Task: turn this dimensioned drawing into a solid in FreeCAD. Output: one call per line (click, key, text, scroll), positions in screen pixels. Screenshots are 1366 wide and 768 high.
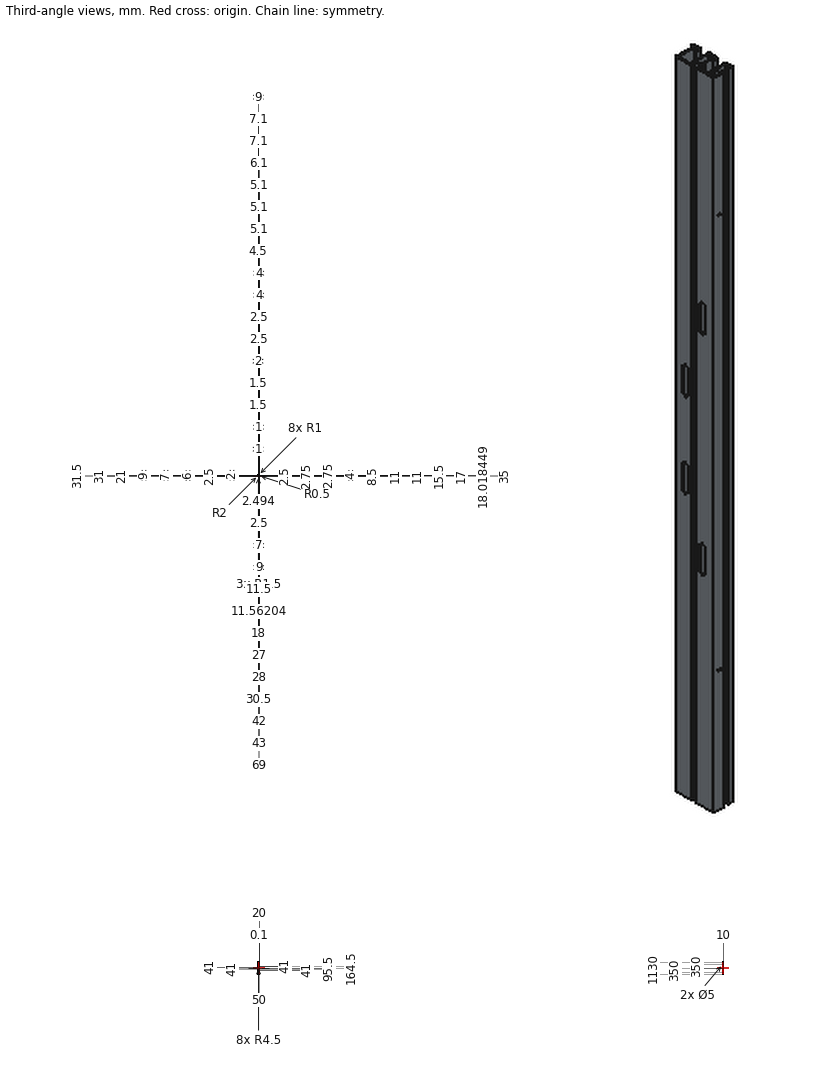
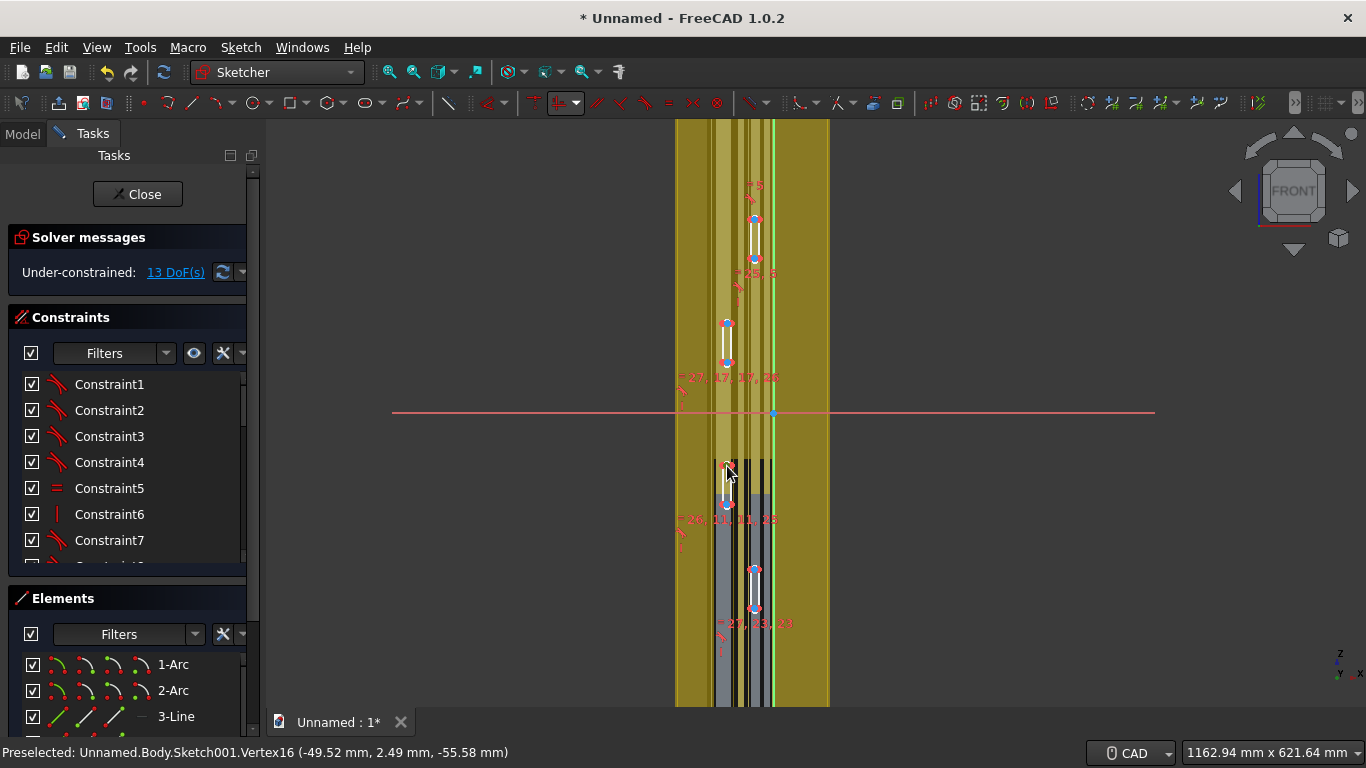
scroll(727, 363, up, 6)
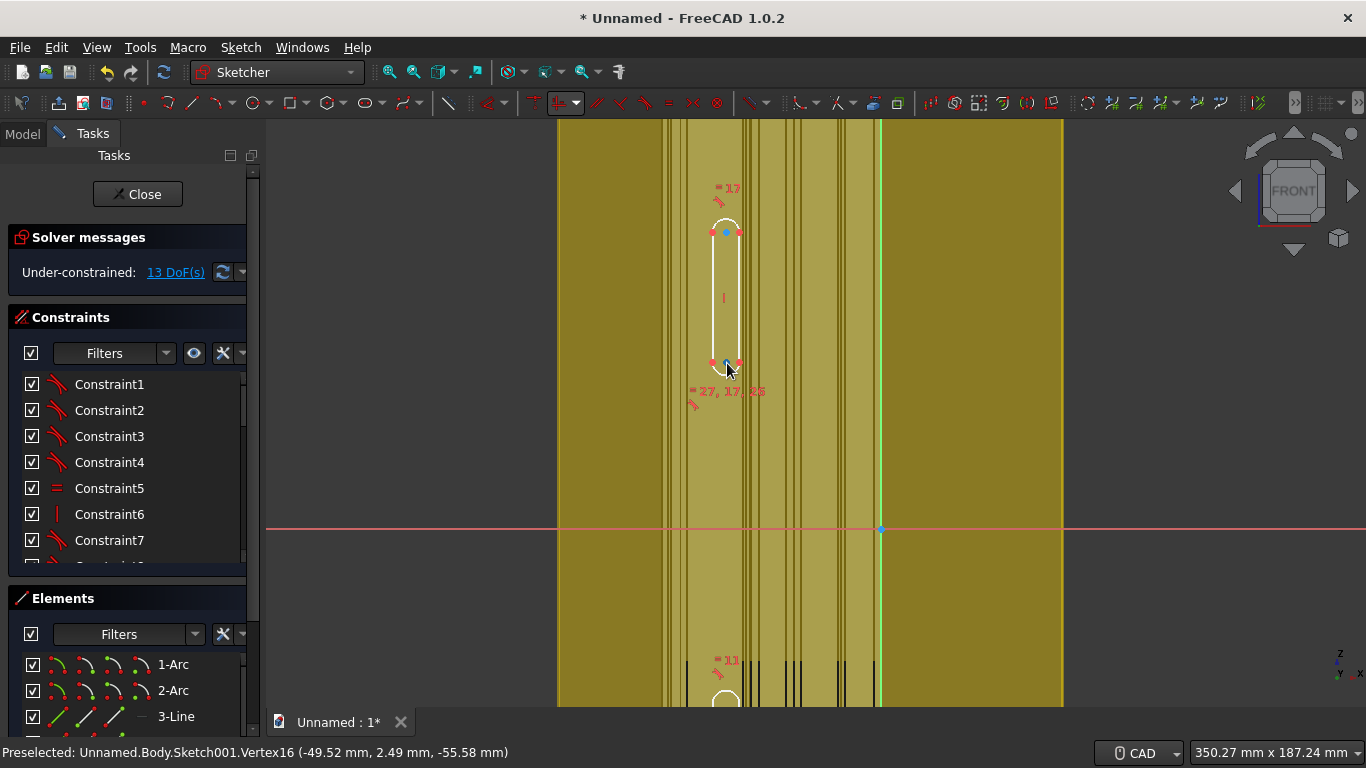
click(726, 362)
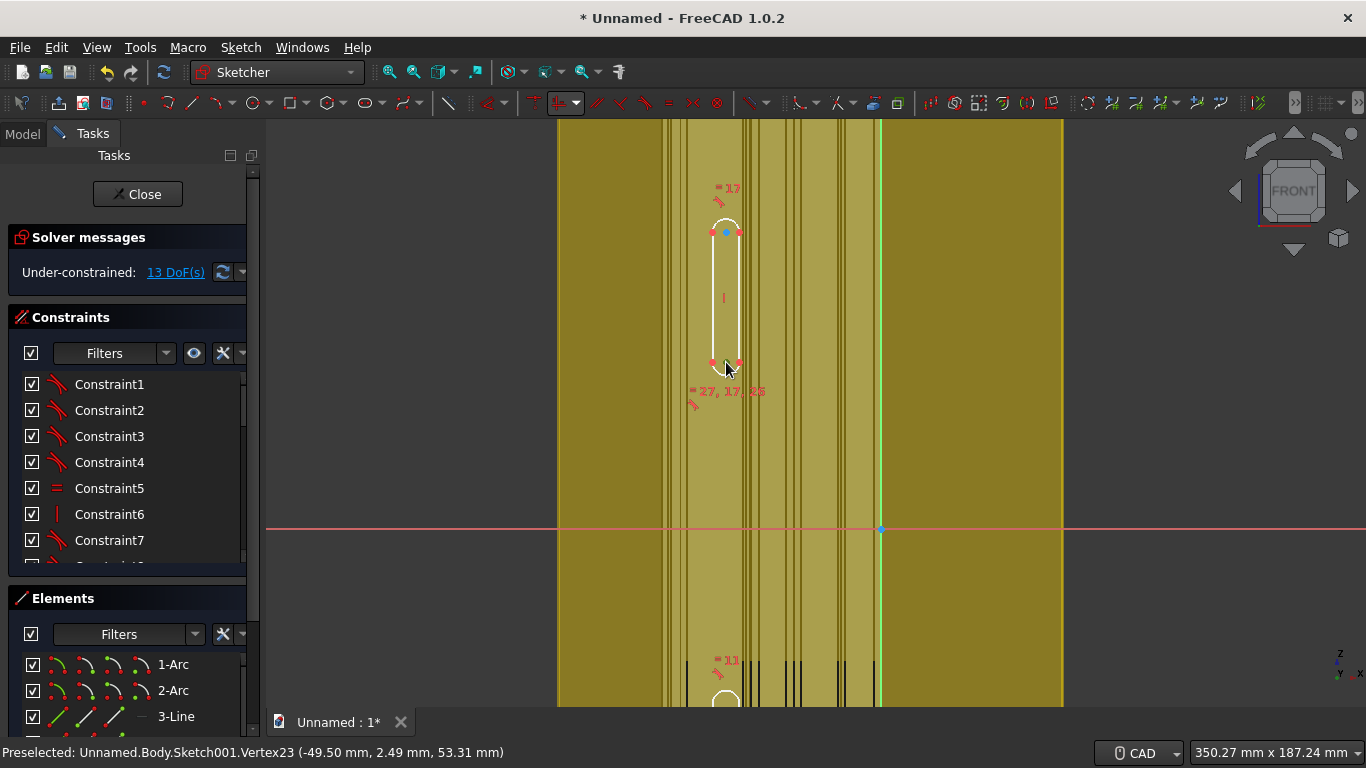
click(359, 529)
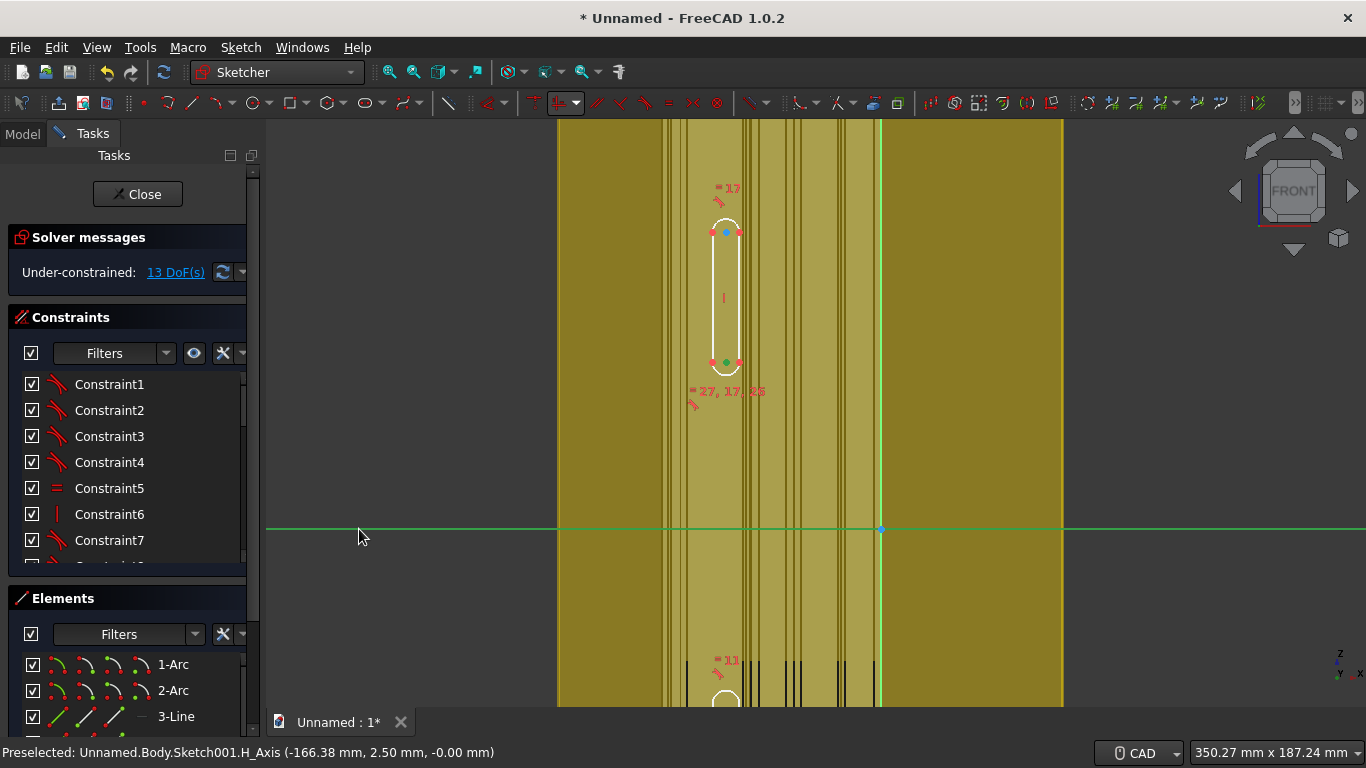
click(694, 104)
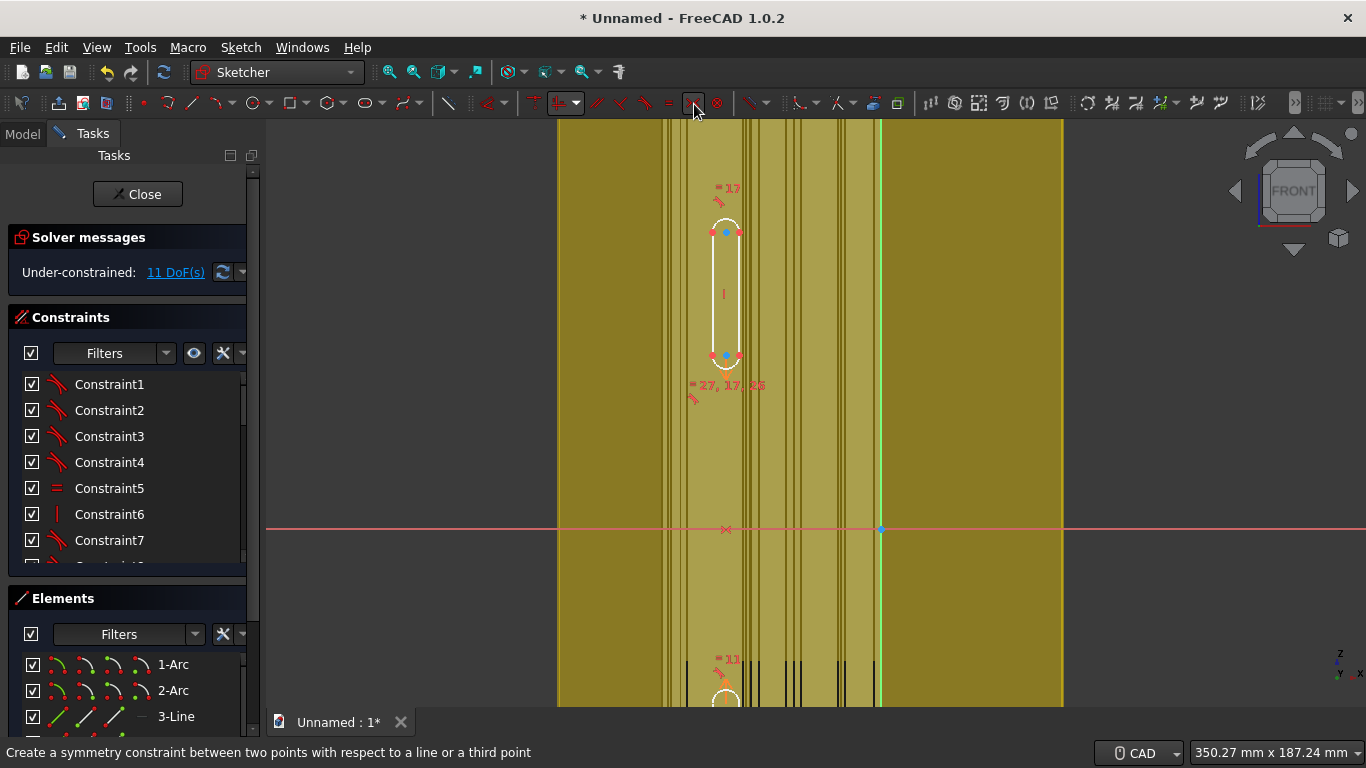
scroll(727, 363, down, 6)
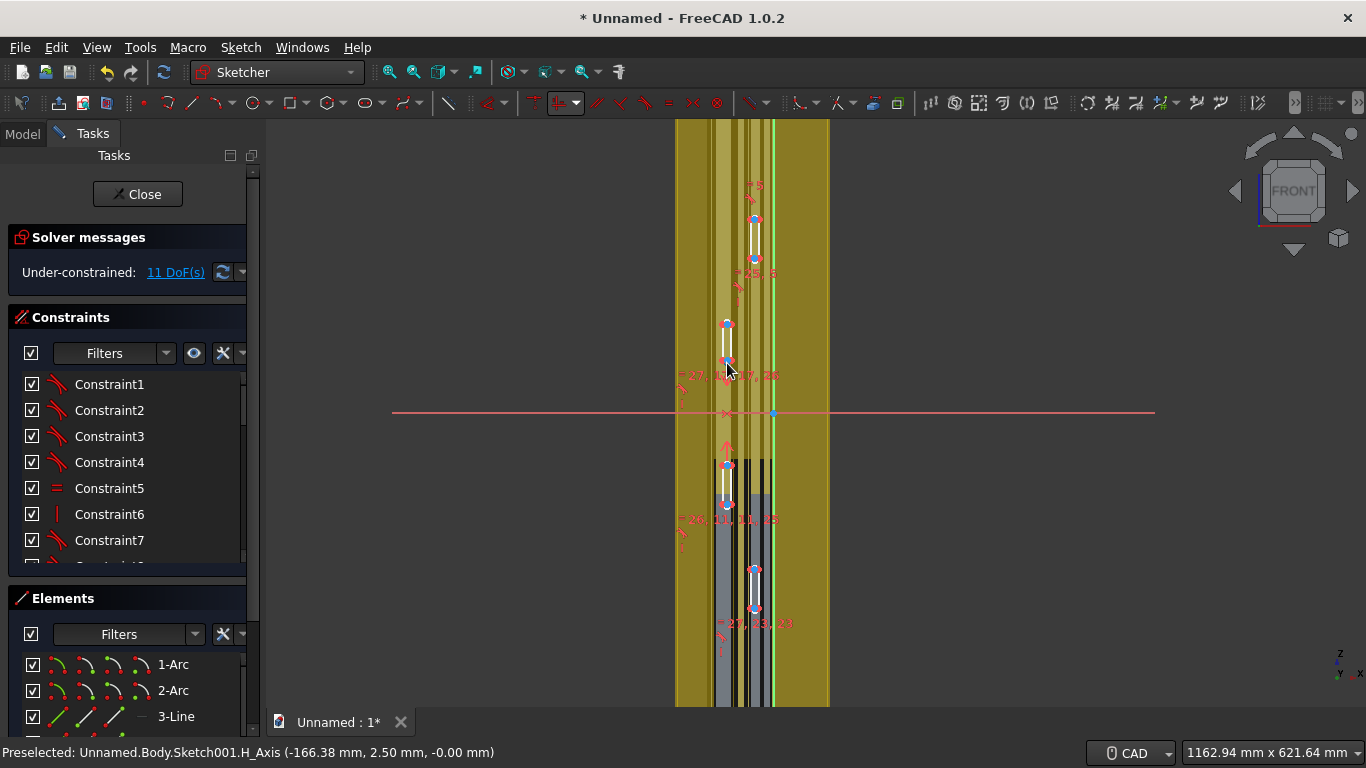
scroll(755, 220, up, 6)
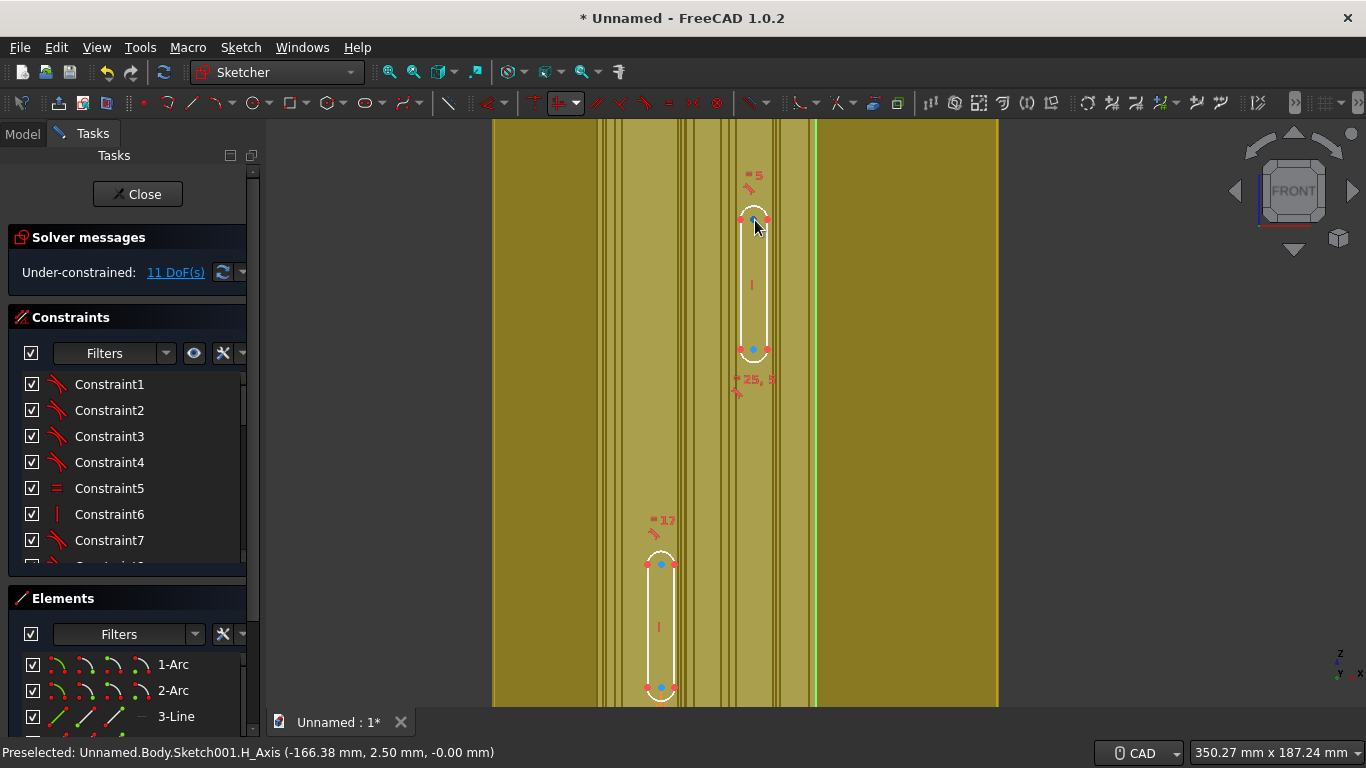
click(754, 220)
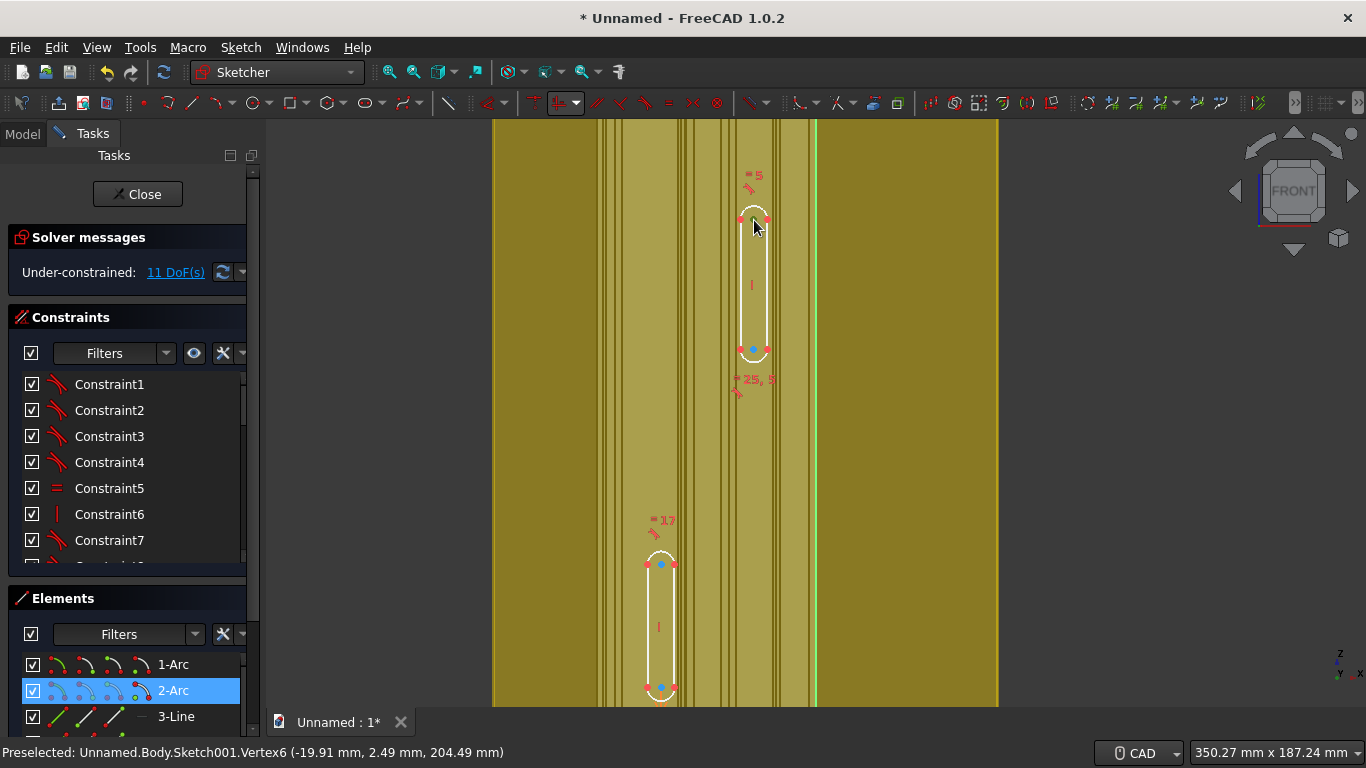
scroll(755, 220, down, 6)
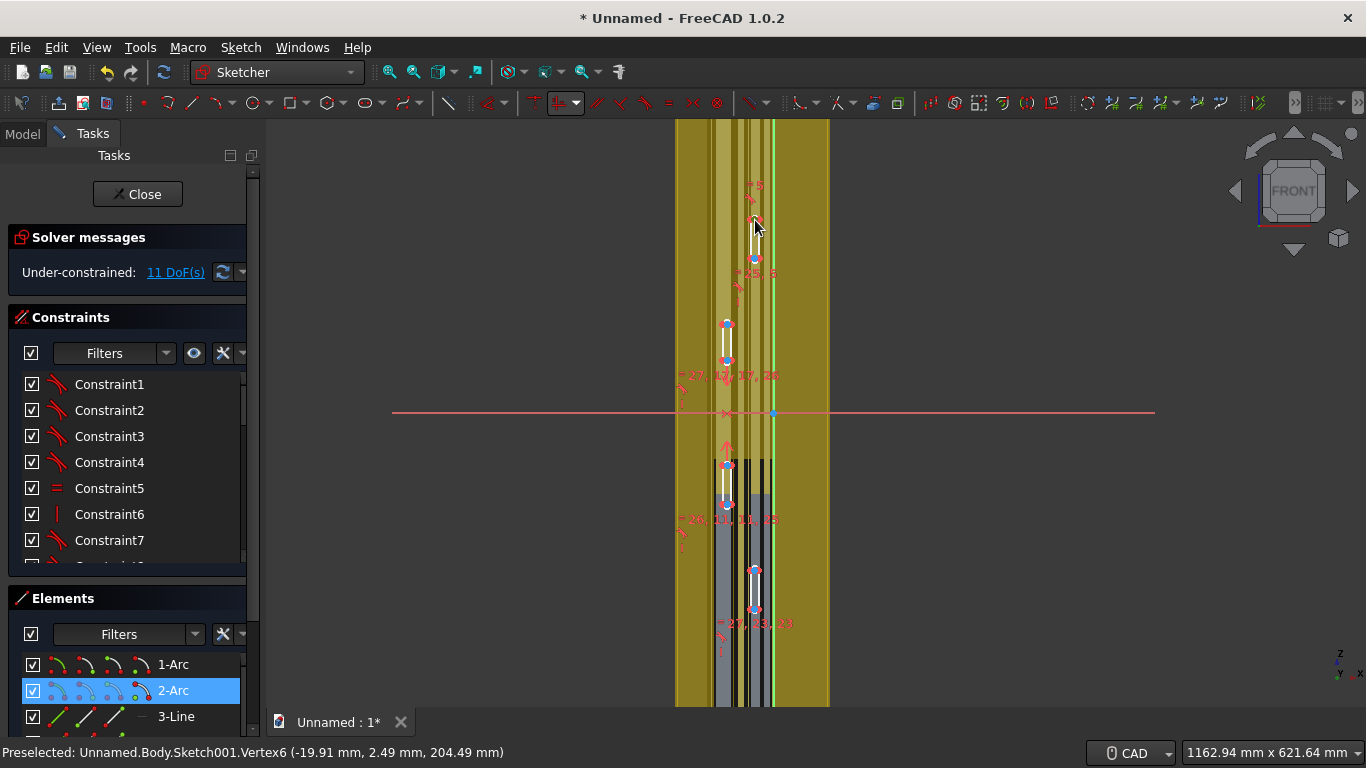
scroll(755, 609, up, 6)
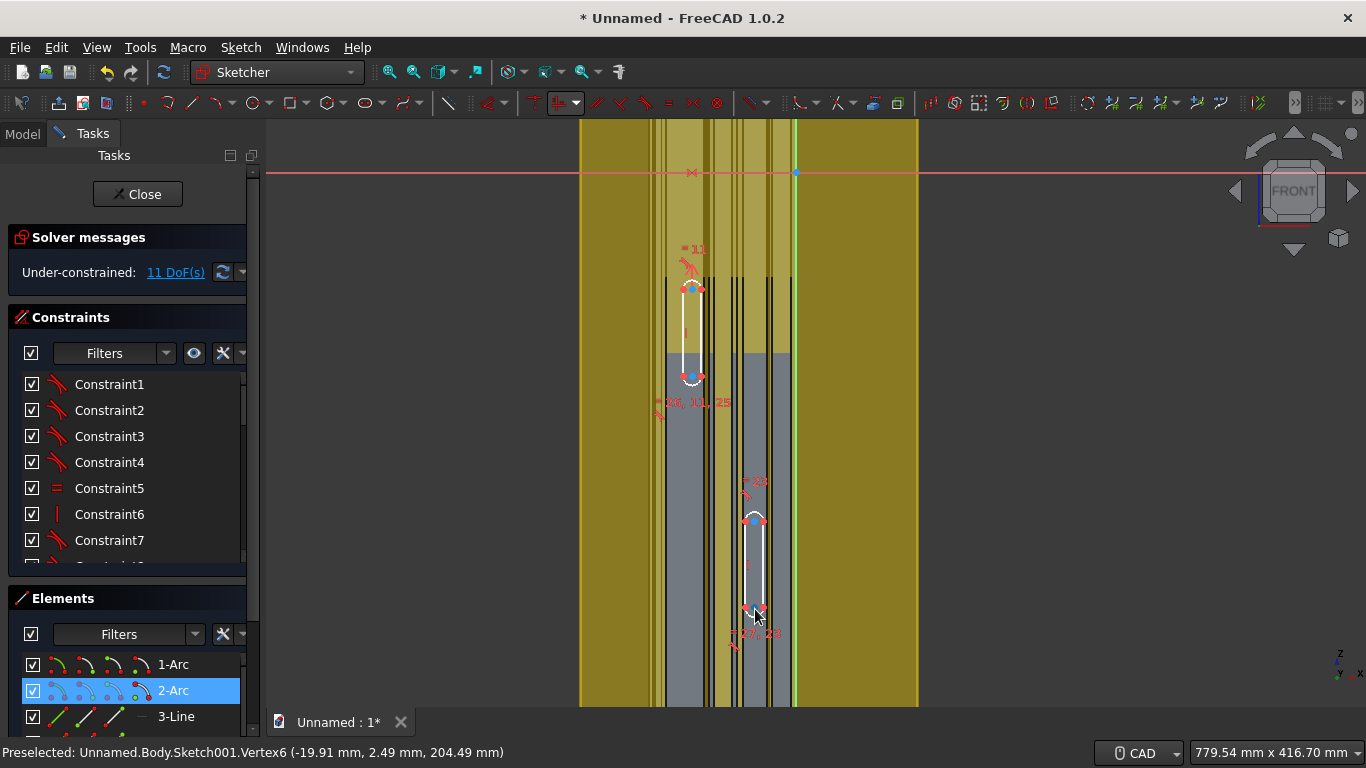
click(754, 607)